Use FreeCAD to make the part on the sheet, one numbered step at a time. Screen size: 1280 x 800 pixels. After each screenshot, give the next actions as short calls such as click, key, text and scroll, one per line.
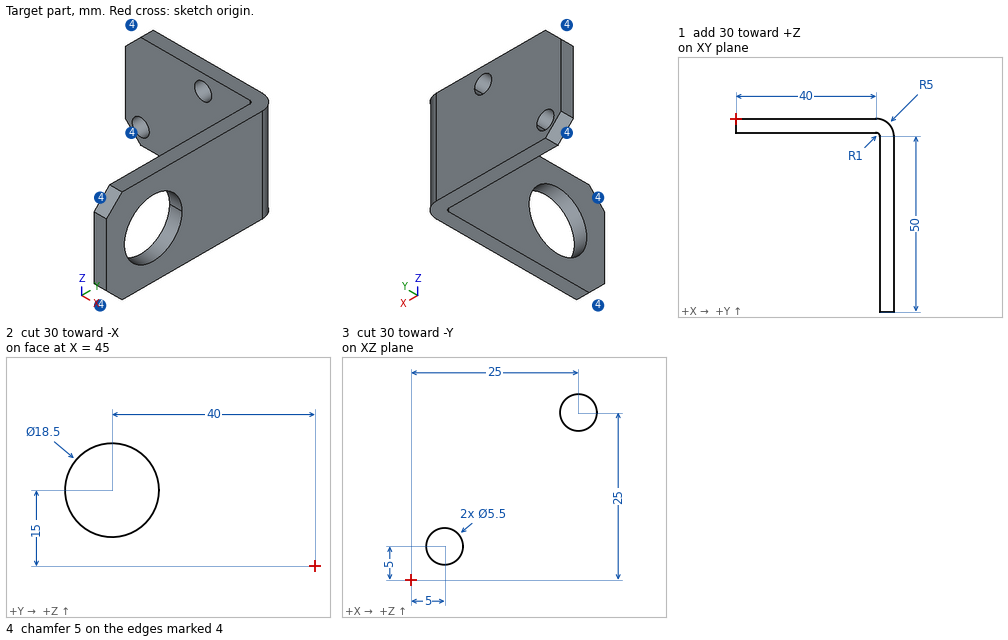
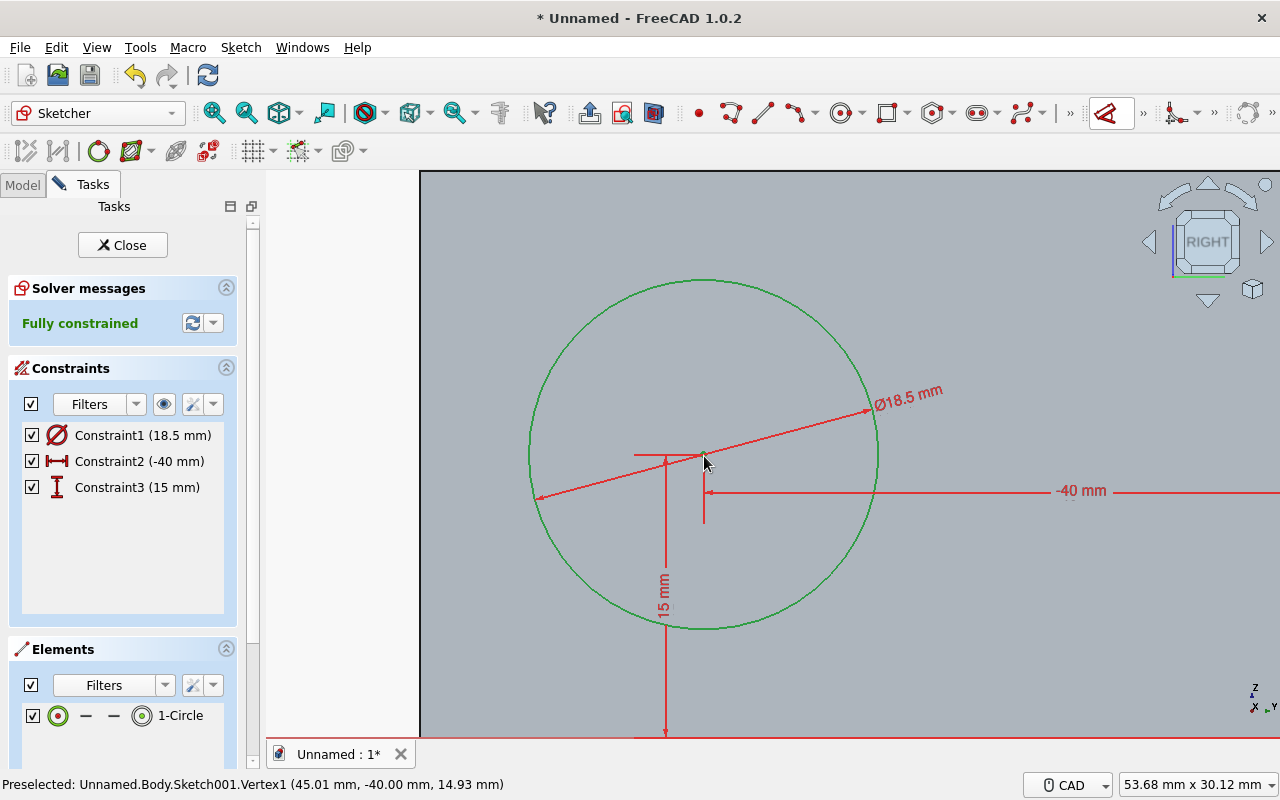
click(123, 245)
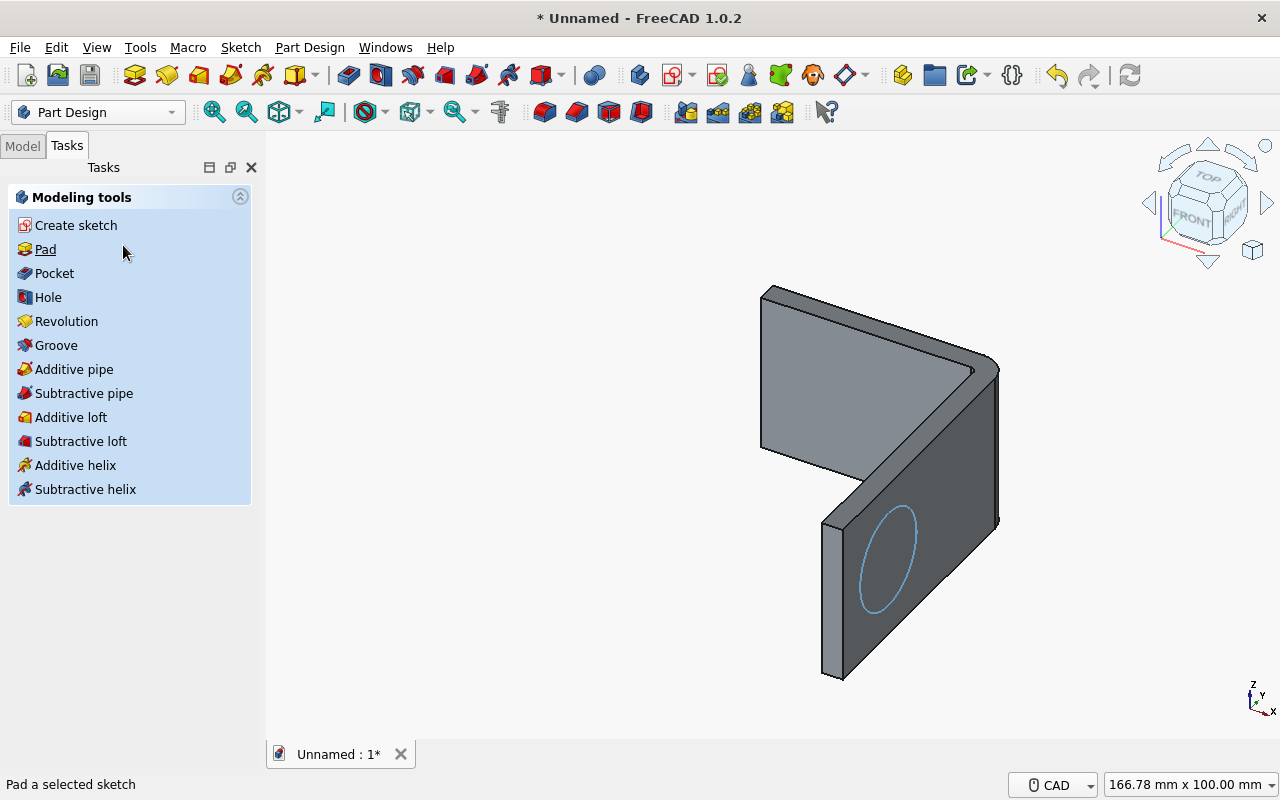
click(350, 76)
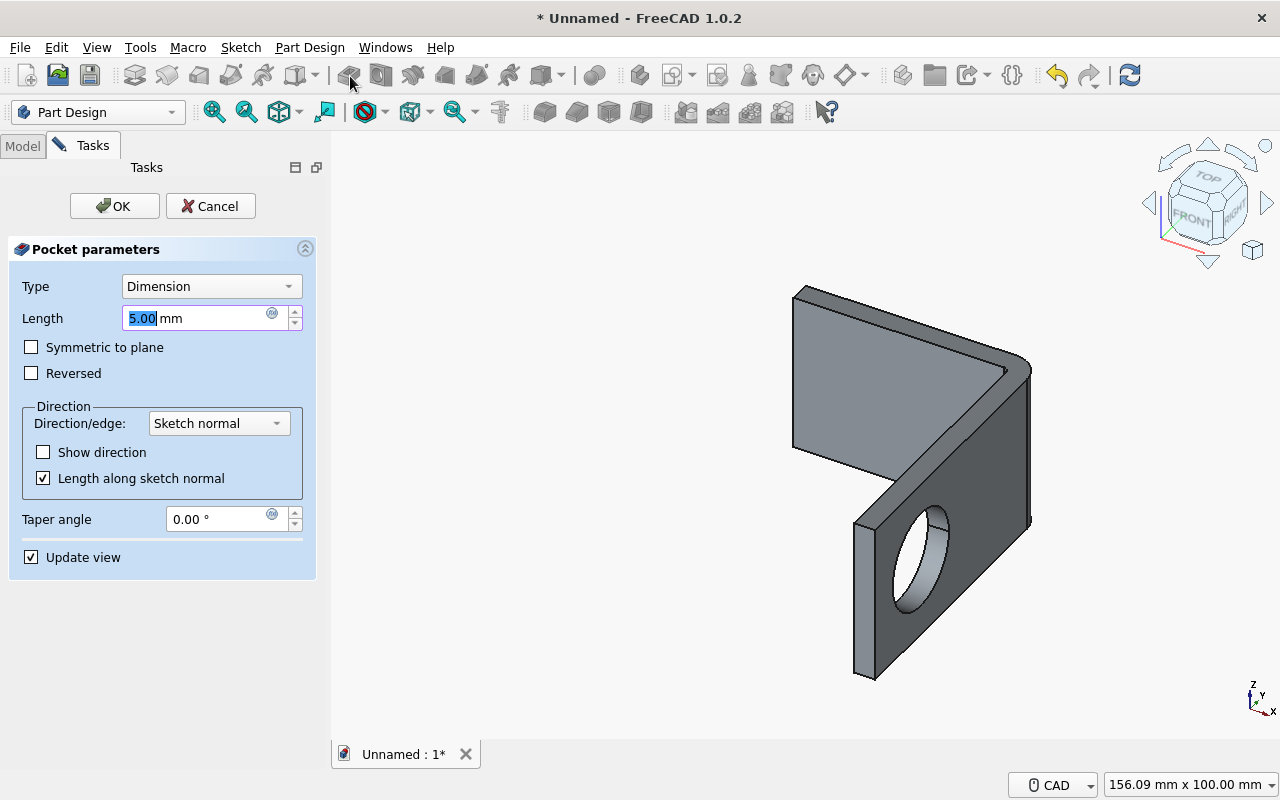
text(30)
key(Tab)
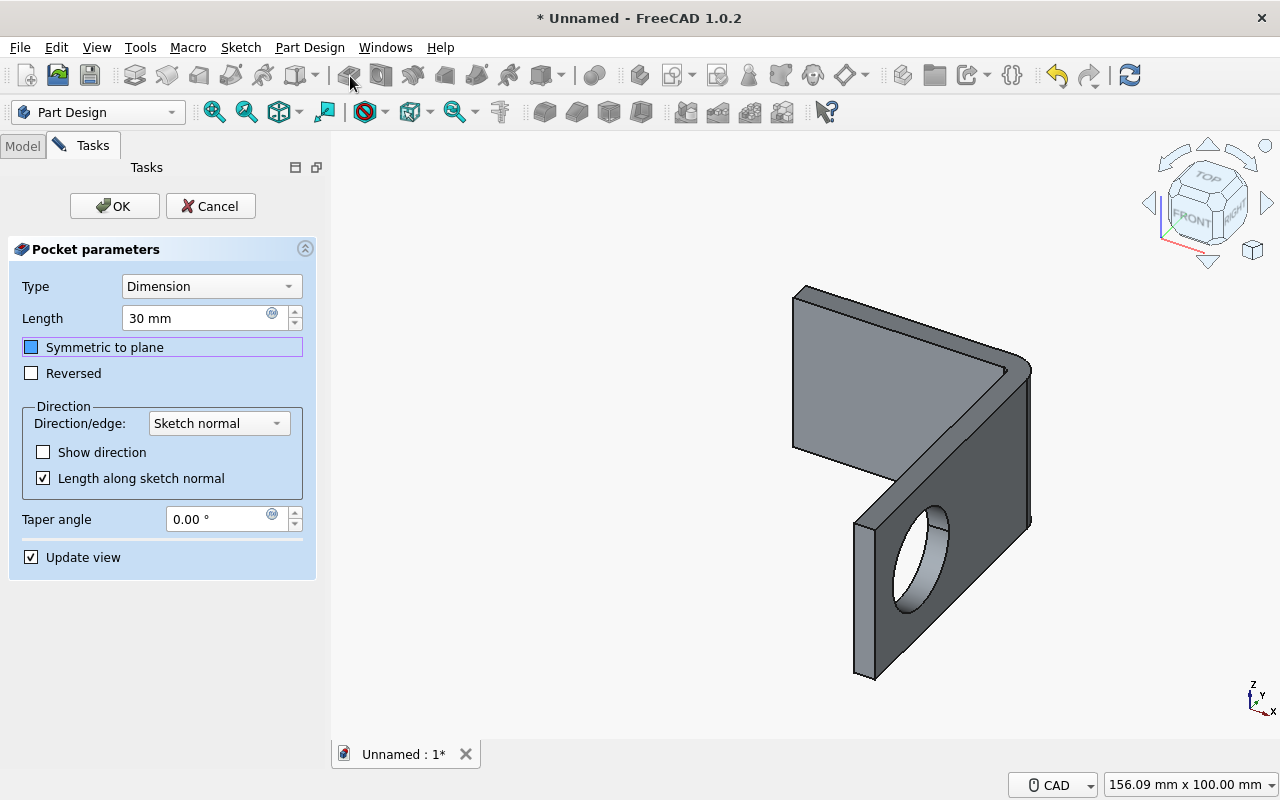
click(115, 206)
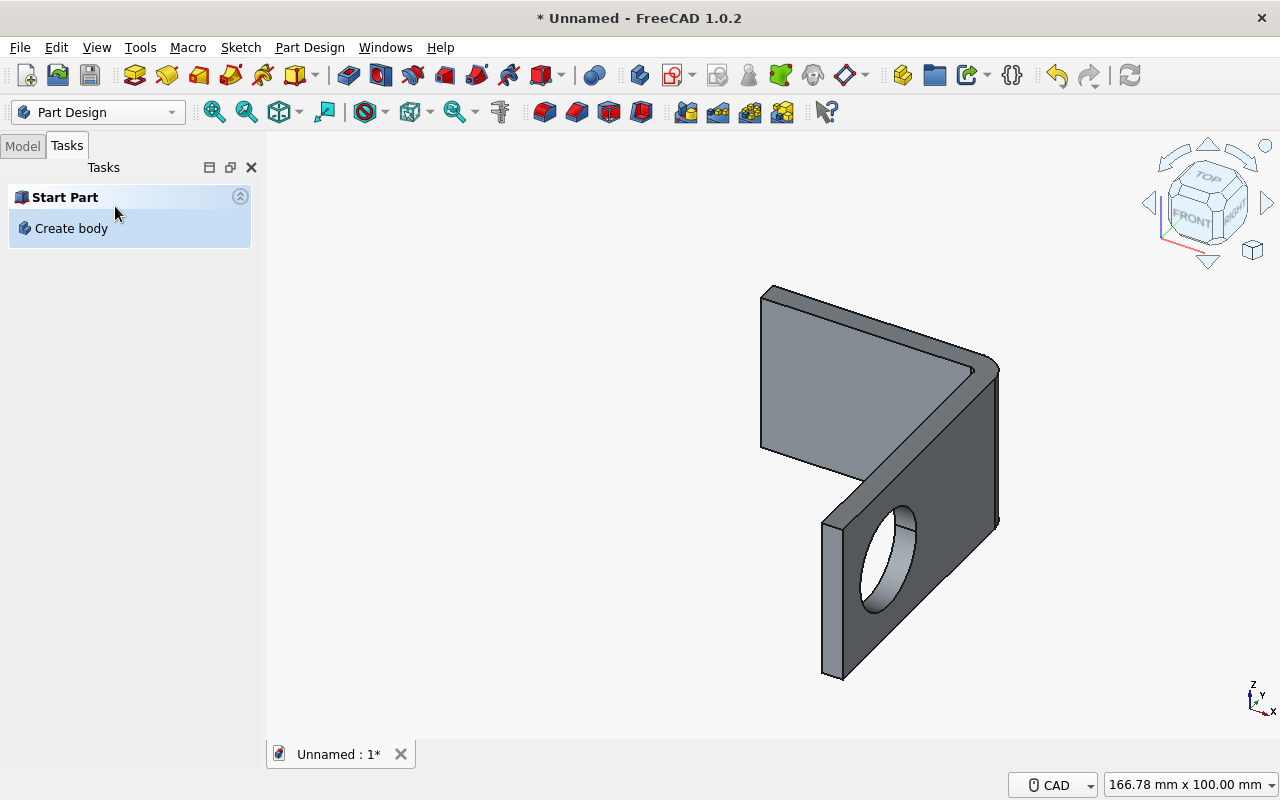
click(672, 76)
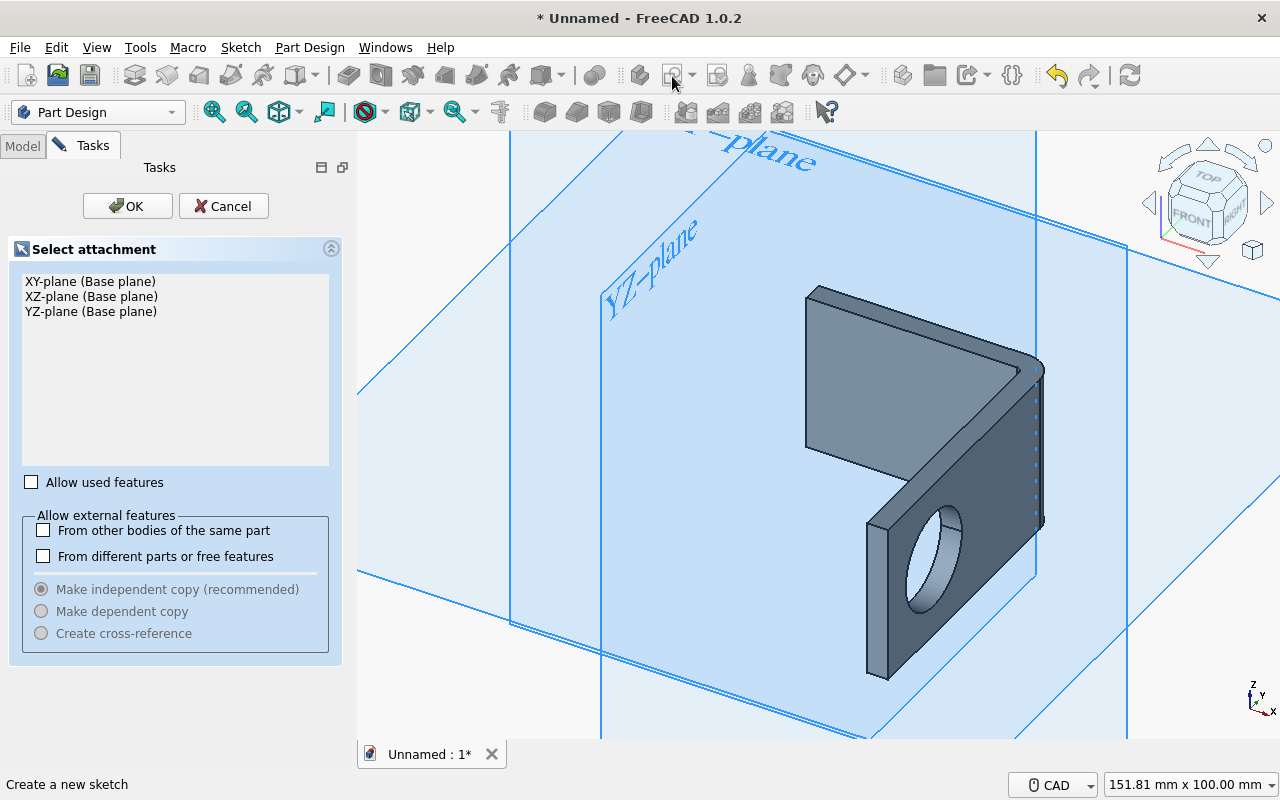
click(82, 296)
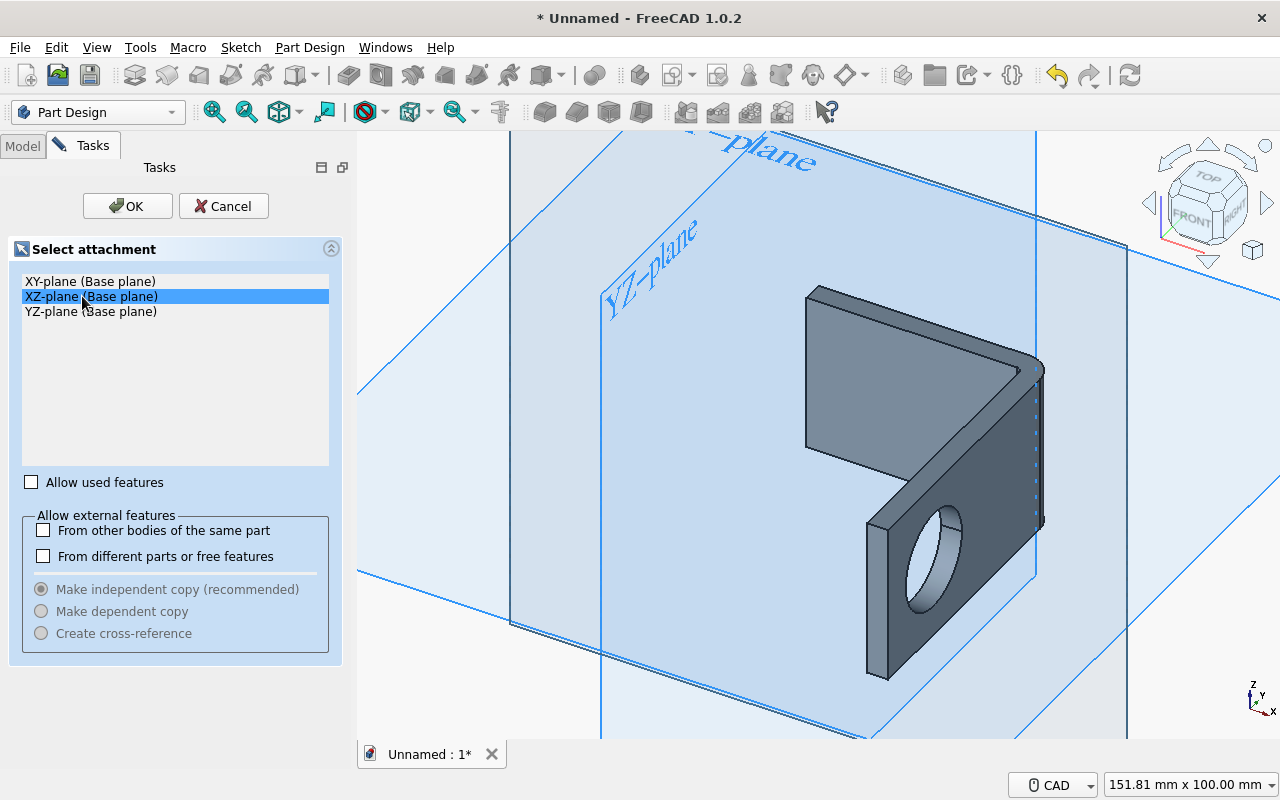
click(128, 206)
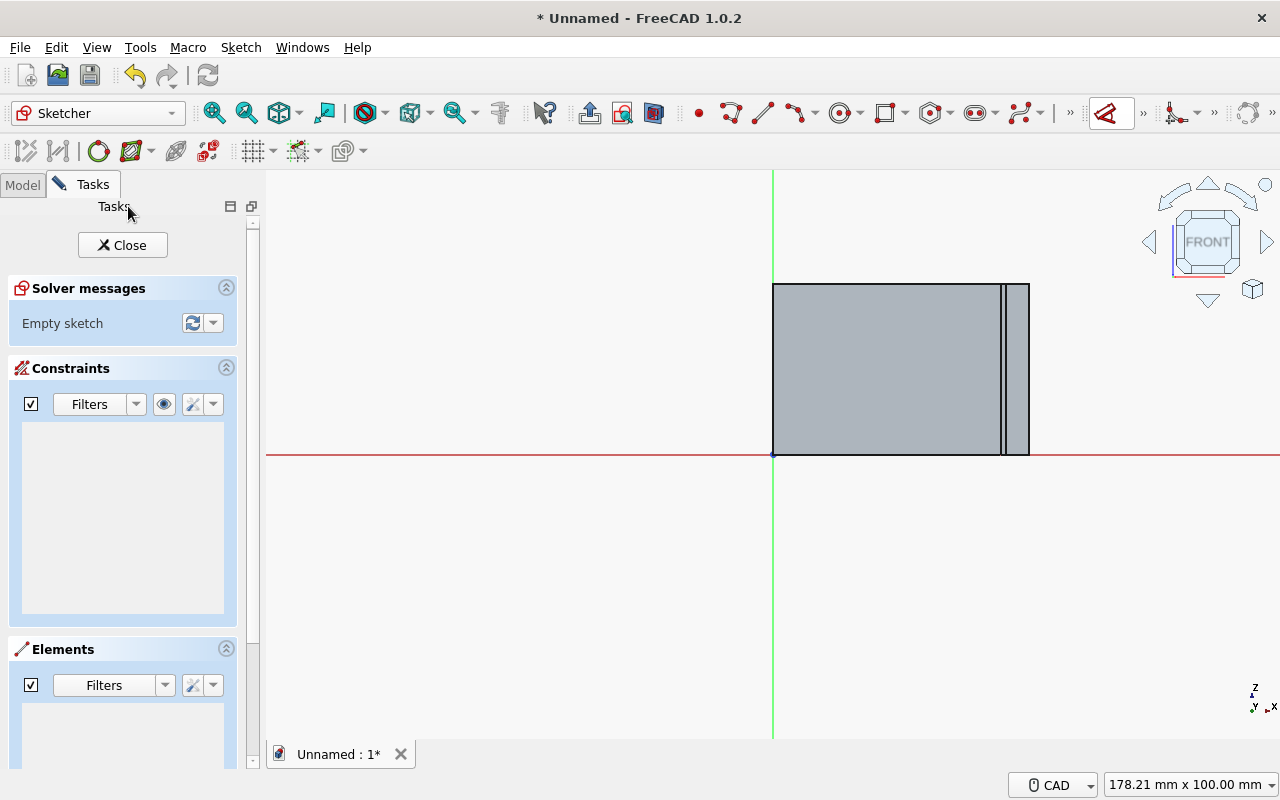
click(654, 114)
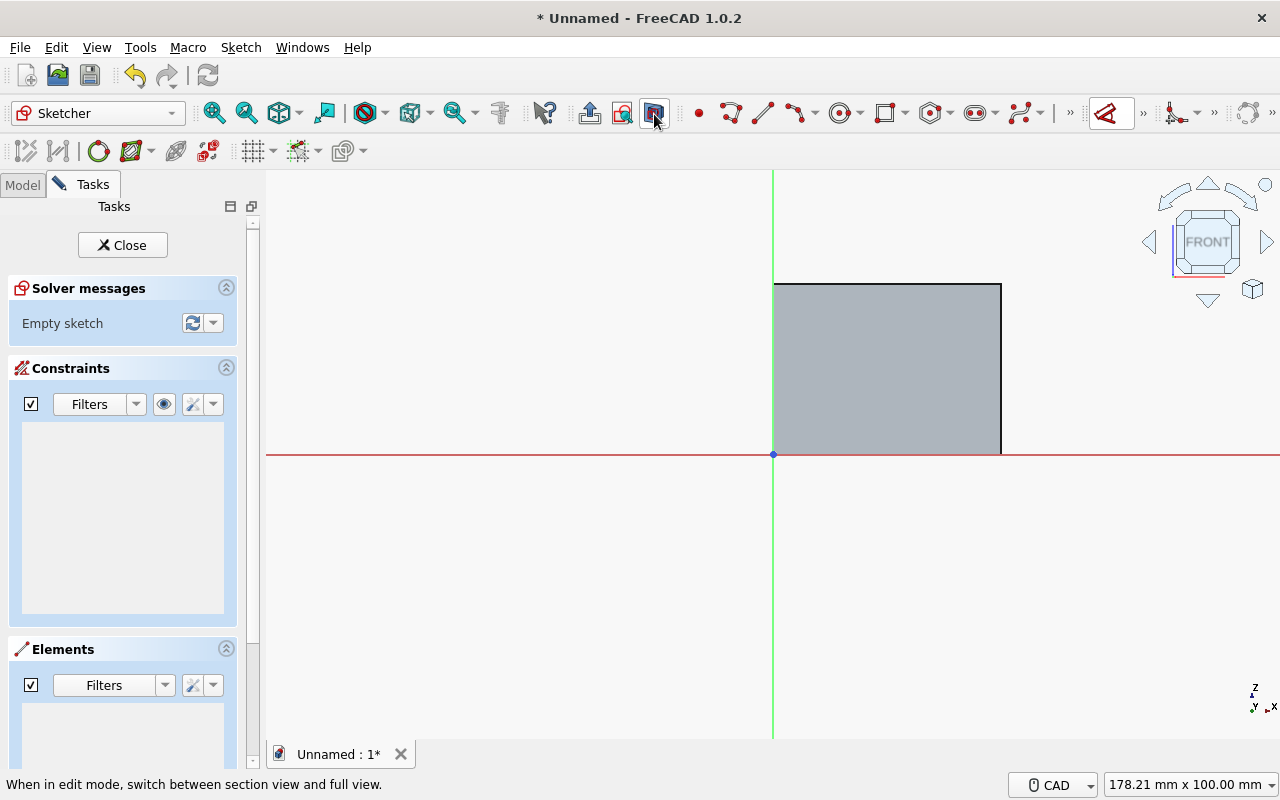
scroll(972, 311, up, 4)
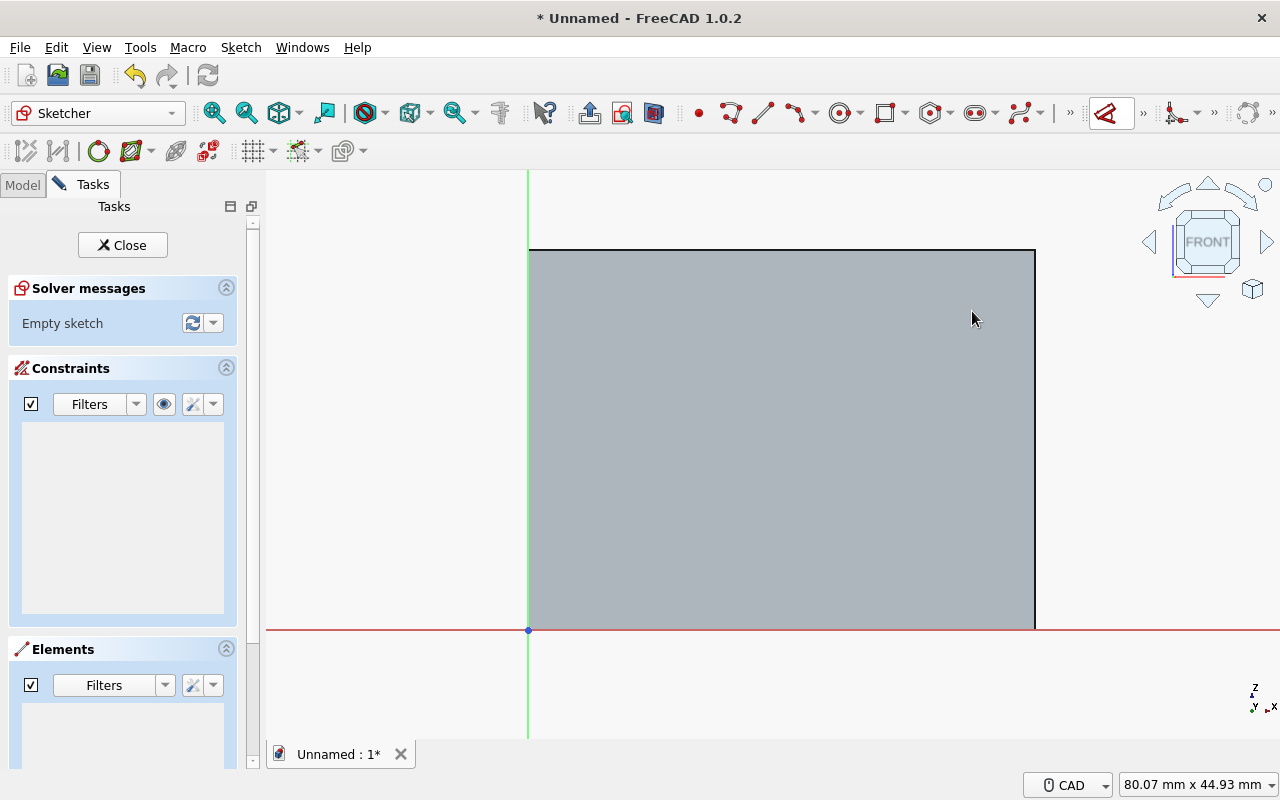
click(840, 114)